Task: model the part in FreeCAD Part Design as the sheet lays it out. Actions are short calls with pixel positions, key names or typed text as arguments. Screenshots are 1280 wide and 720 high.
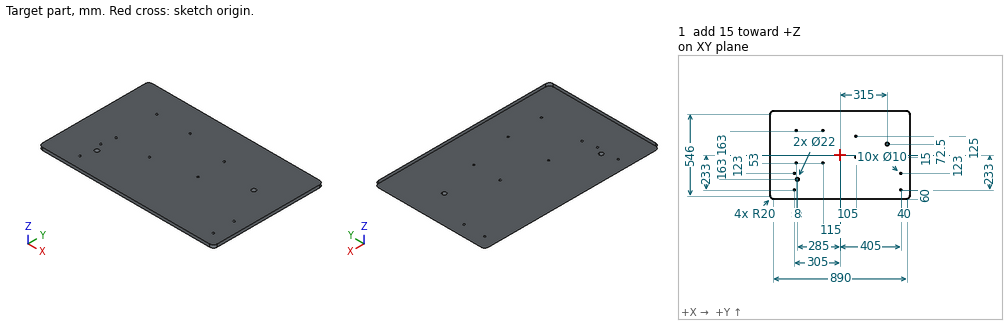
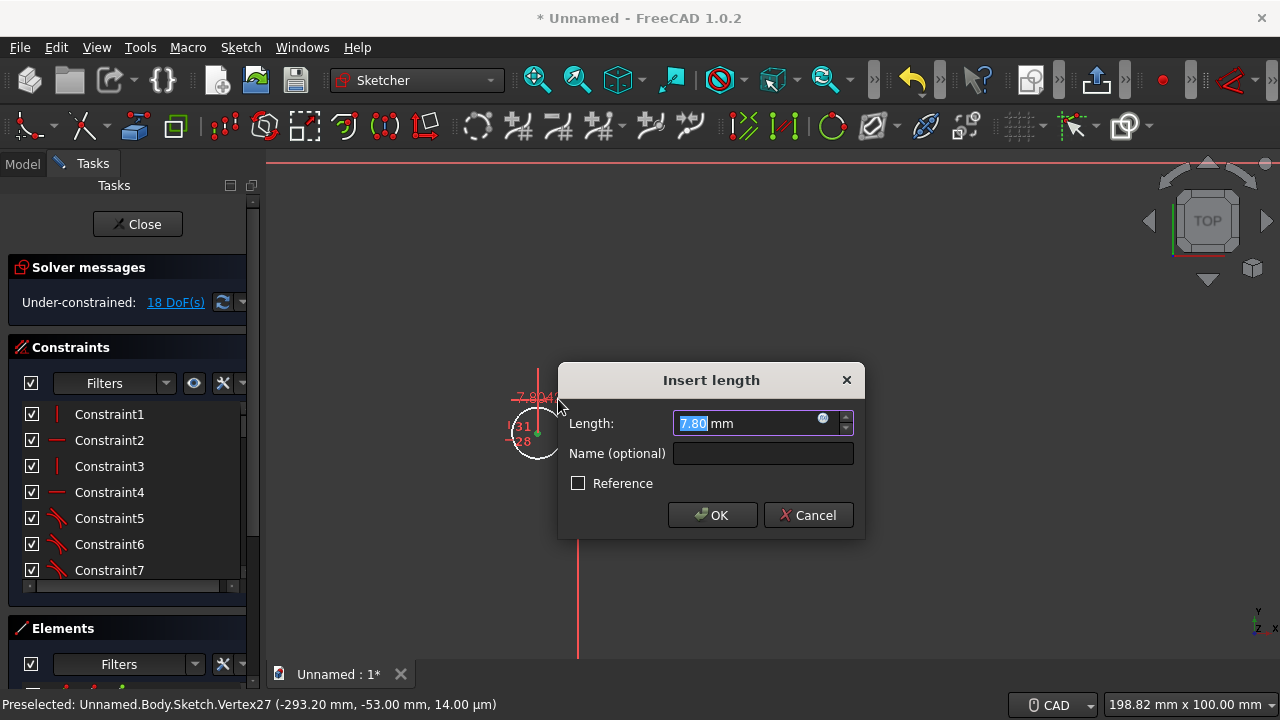
text(8)
key(Return)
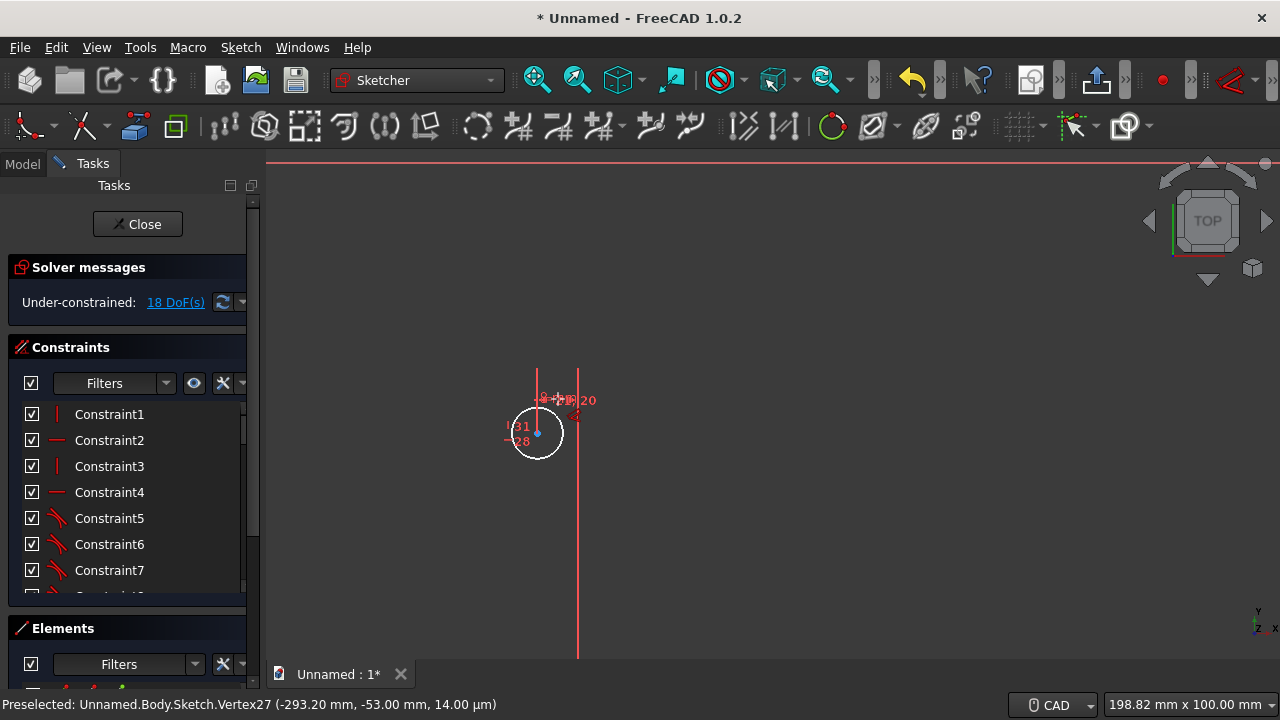
scroll(539, 434, down, 11)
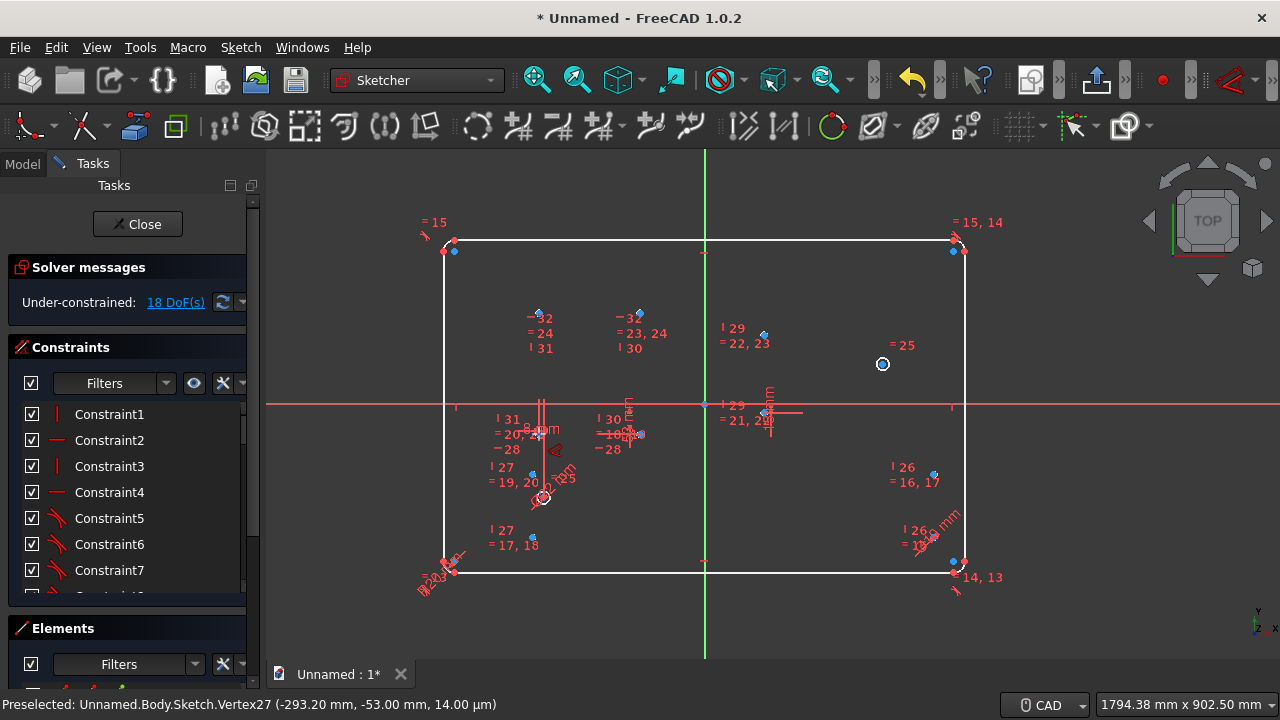
click(444, 345)
click(410, 335)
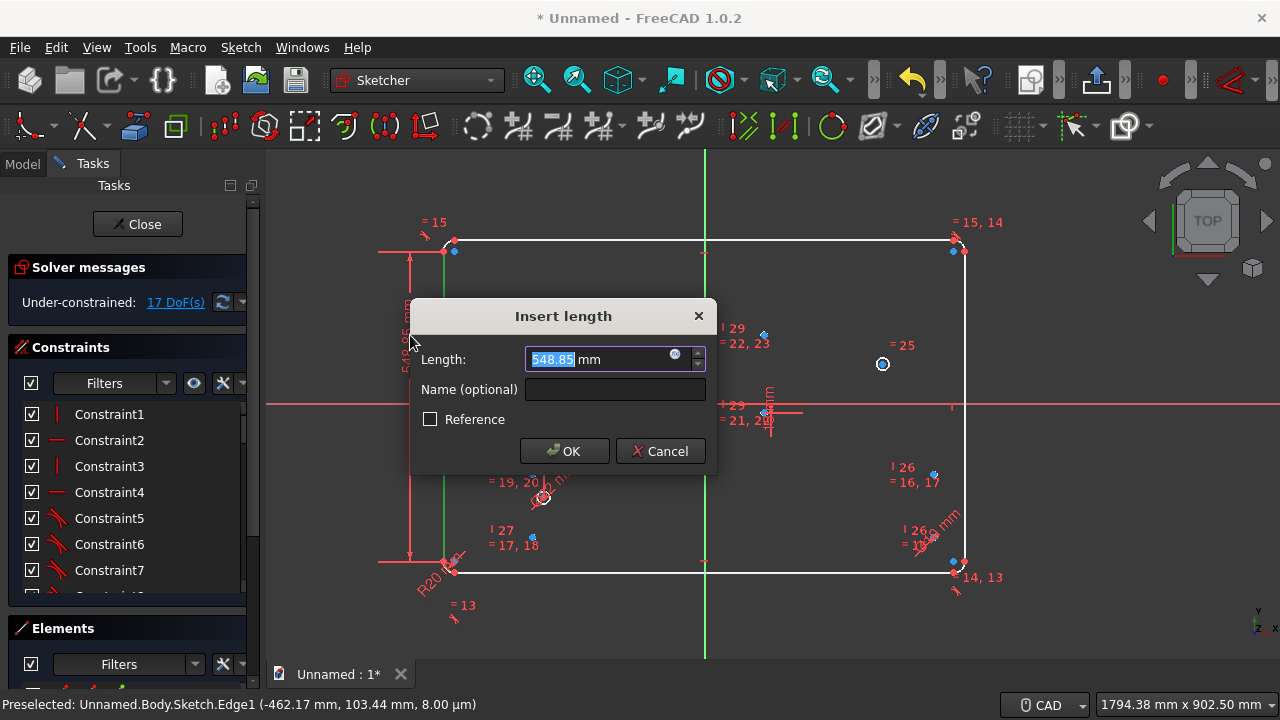
text(546)
key(Return)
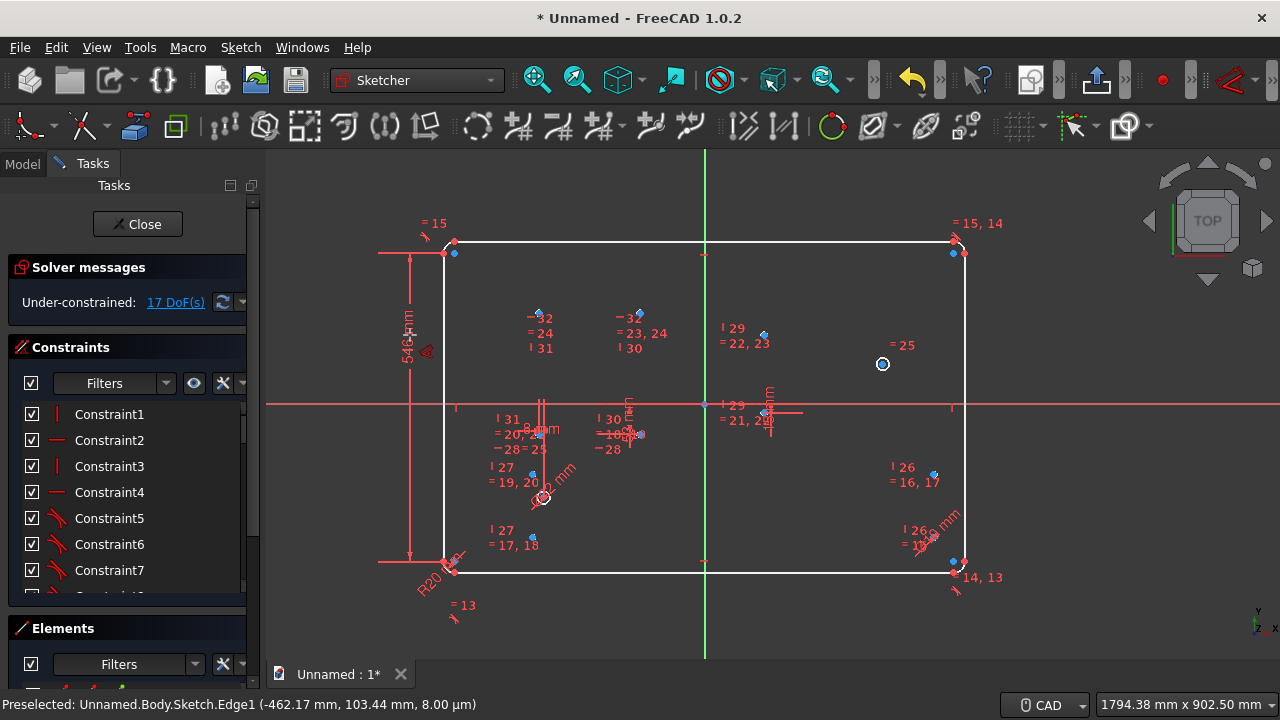
click(605, 573)
click(590, 607)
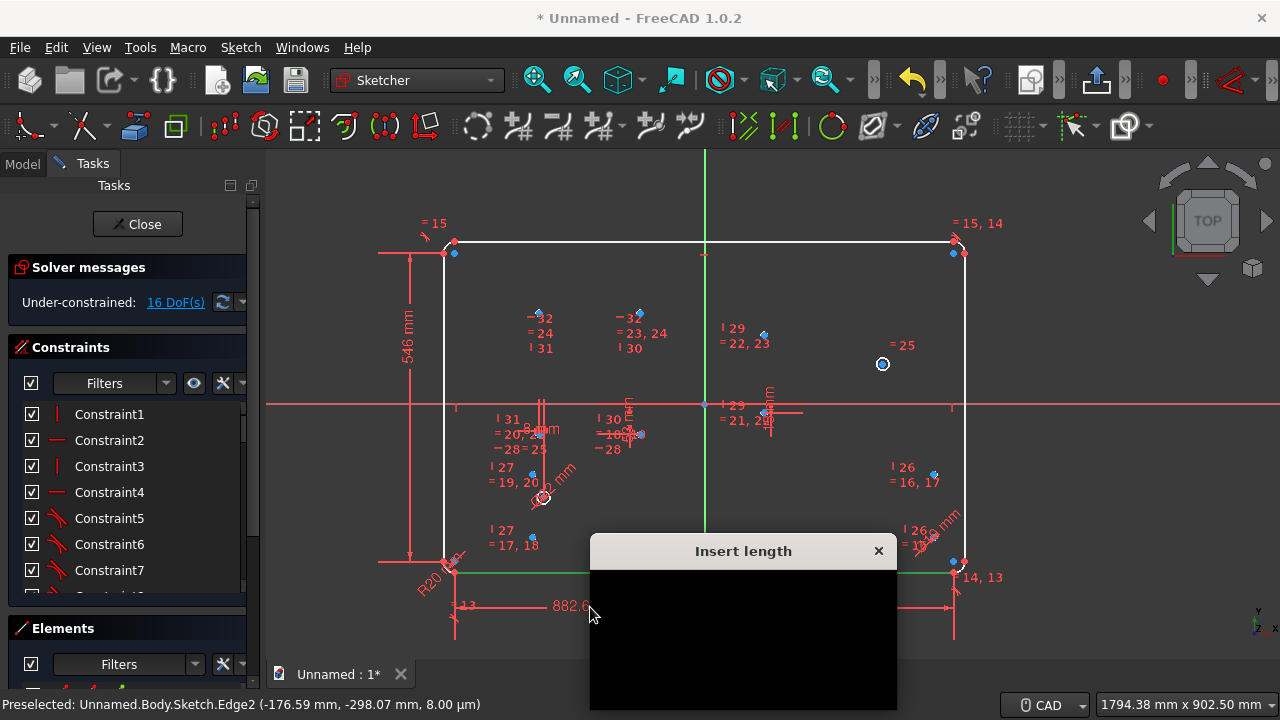
text(890)
key(Return)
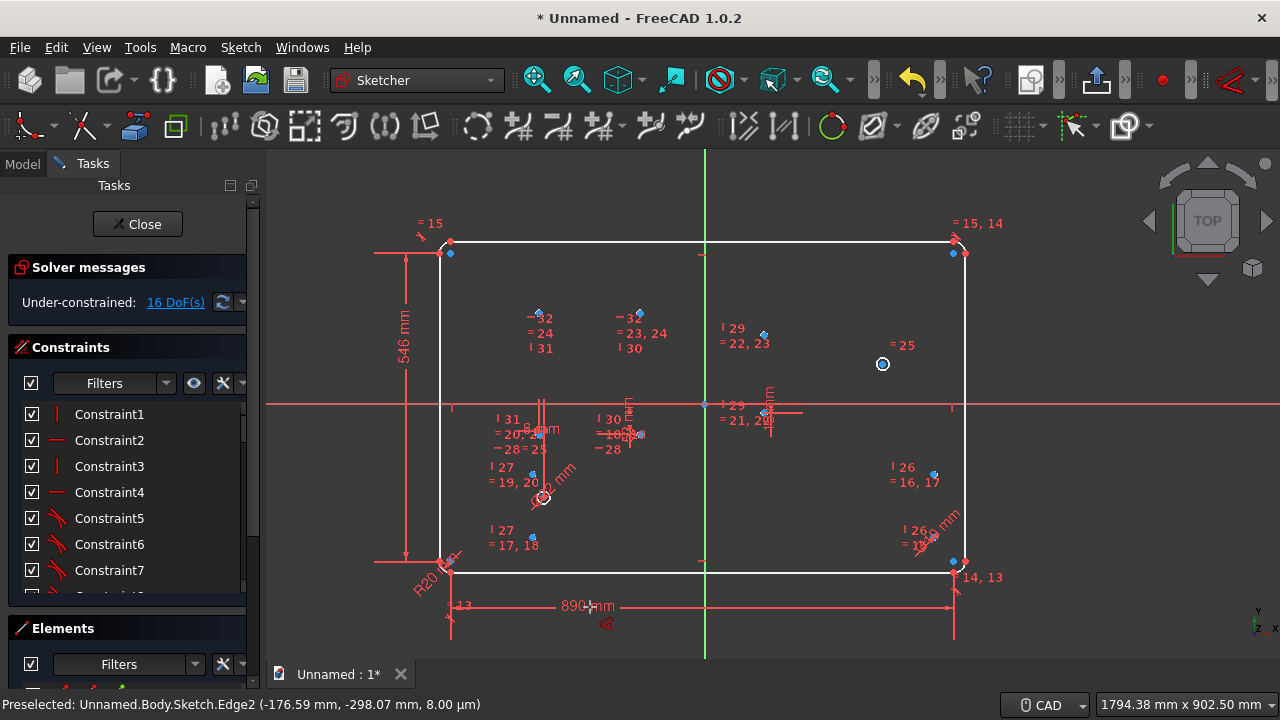
click(934, 537)
click(819, 370)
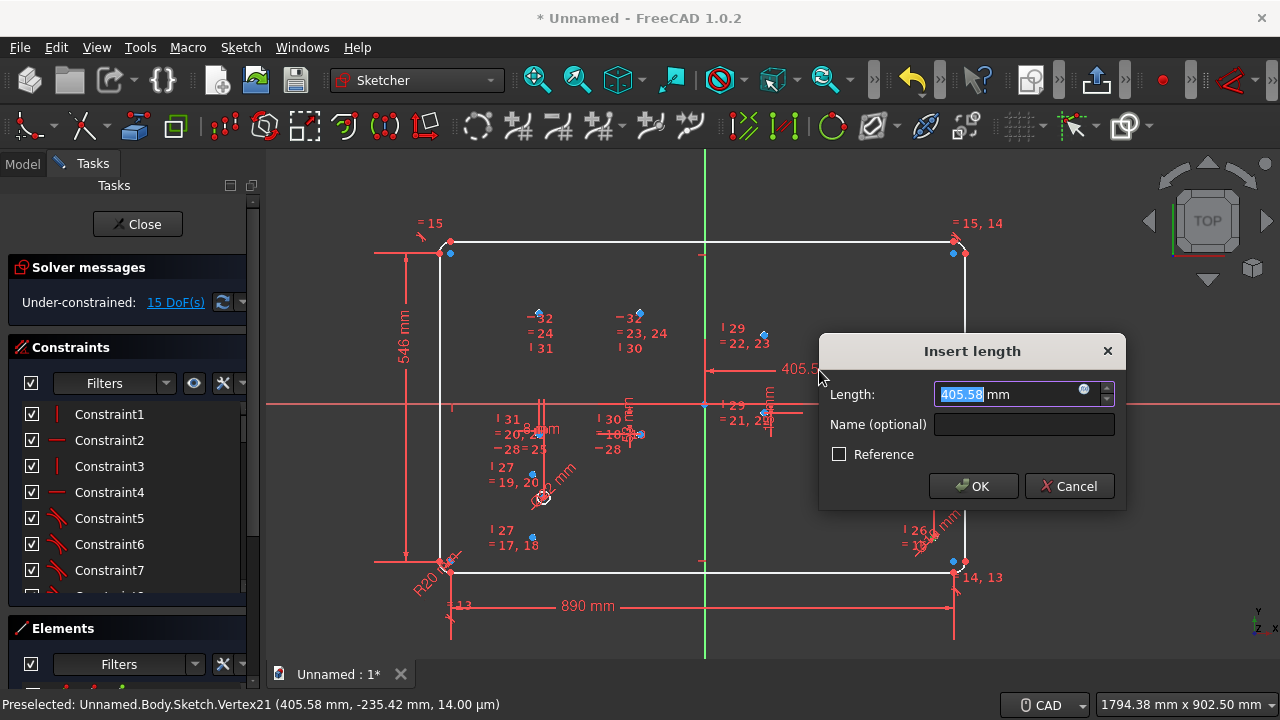
text(405)
key(Return)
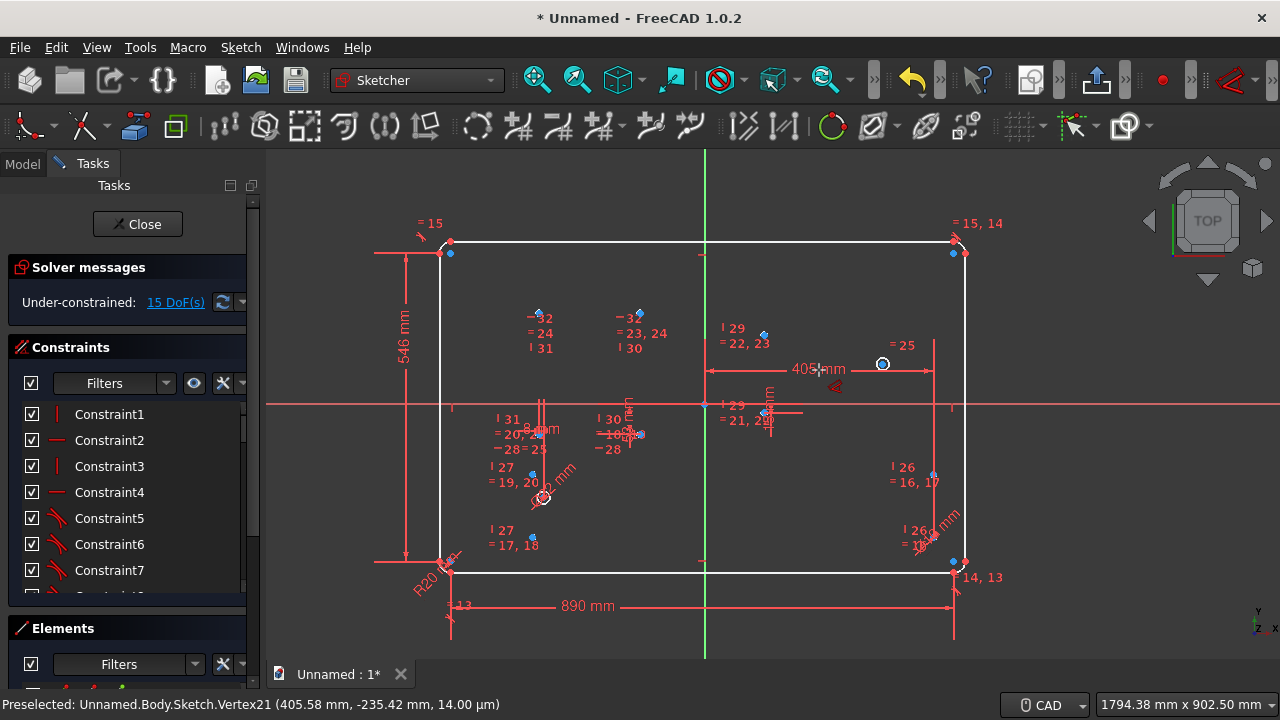
click(934, 537)
click(671, 471)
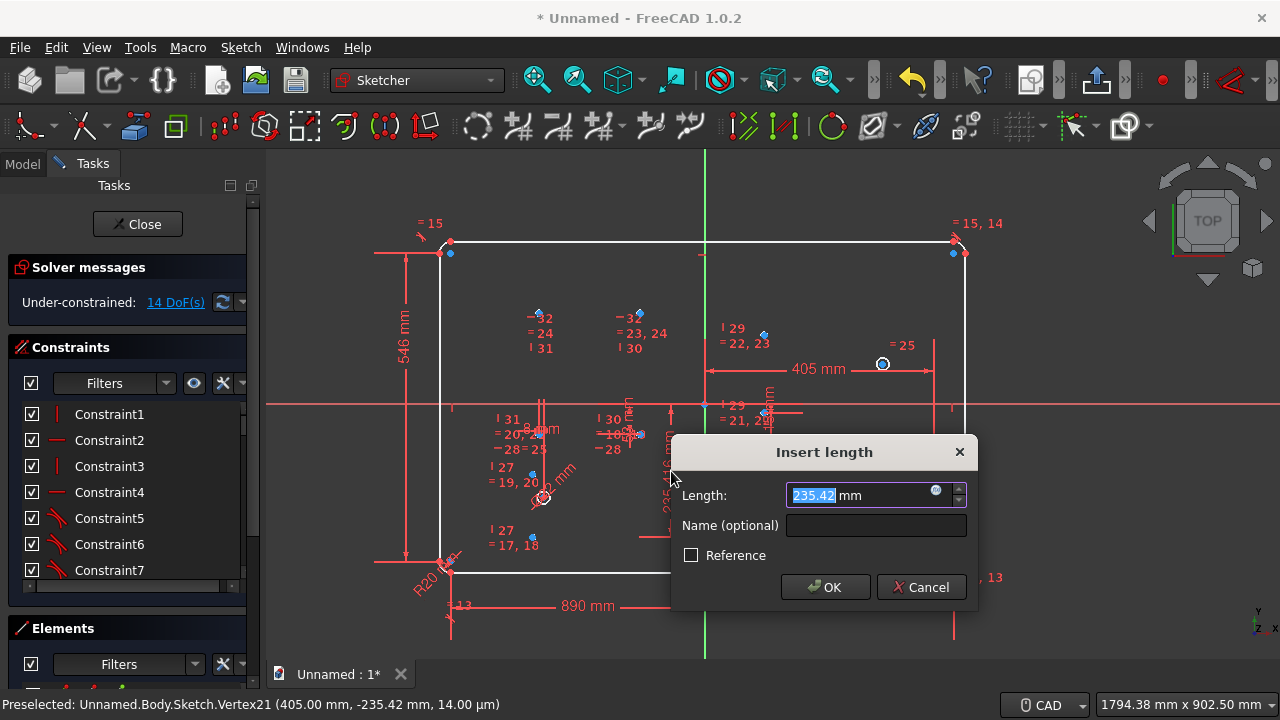
text(233)
key(Return)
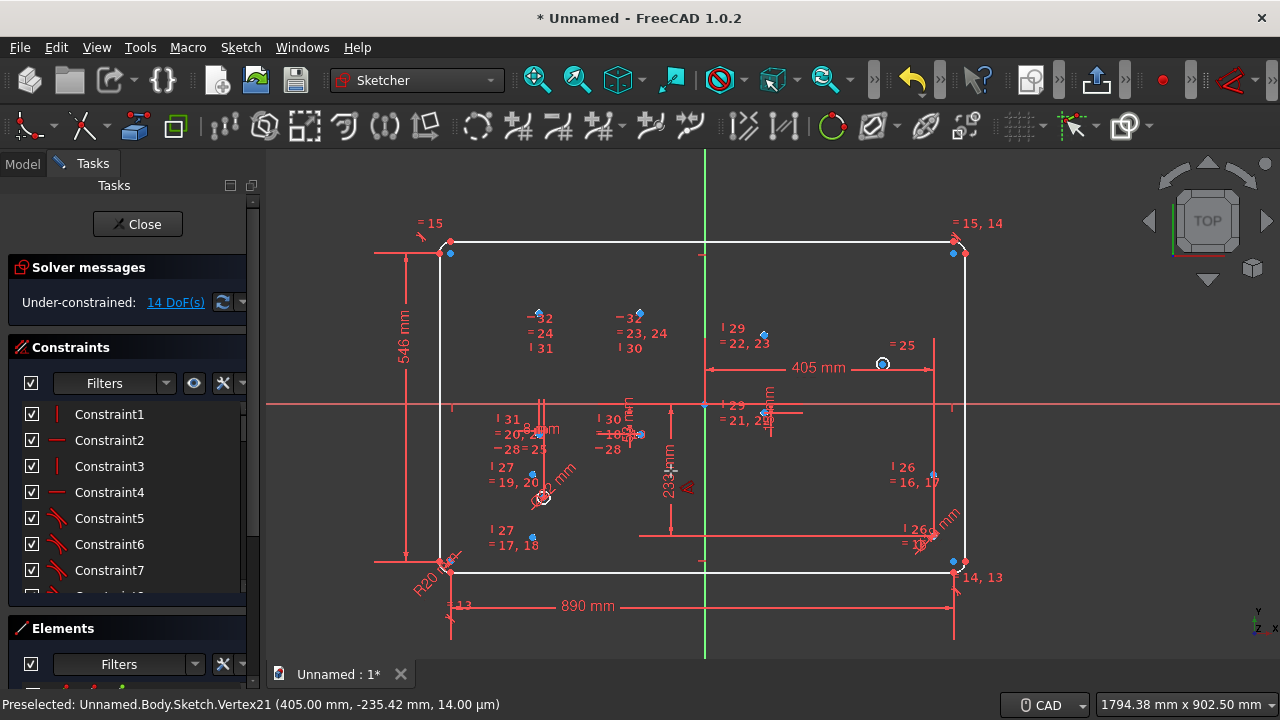
click(934, 475)
click(992, 440)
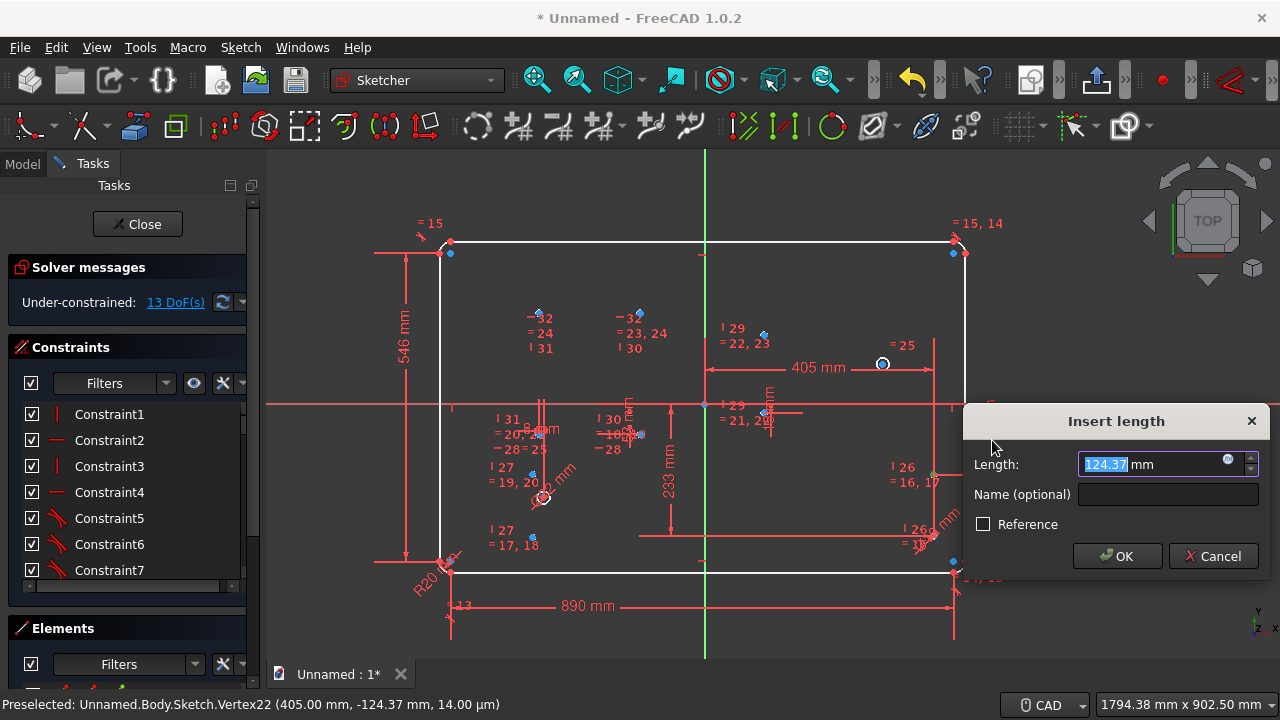
text(123)
key(Return)